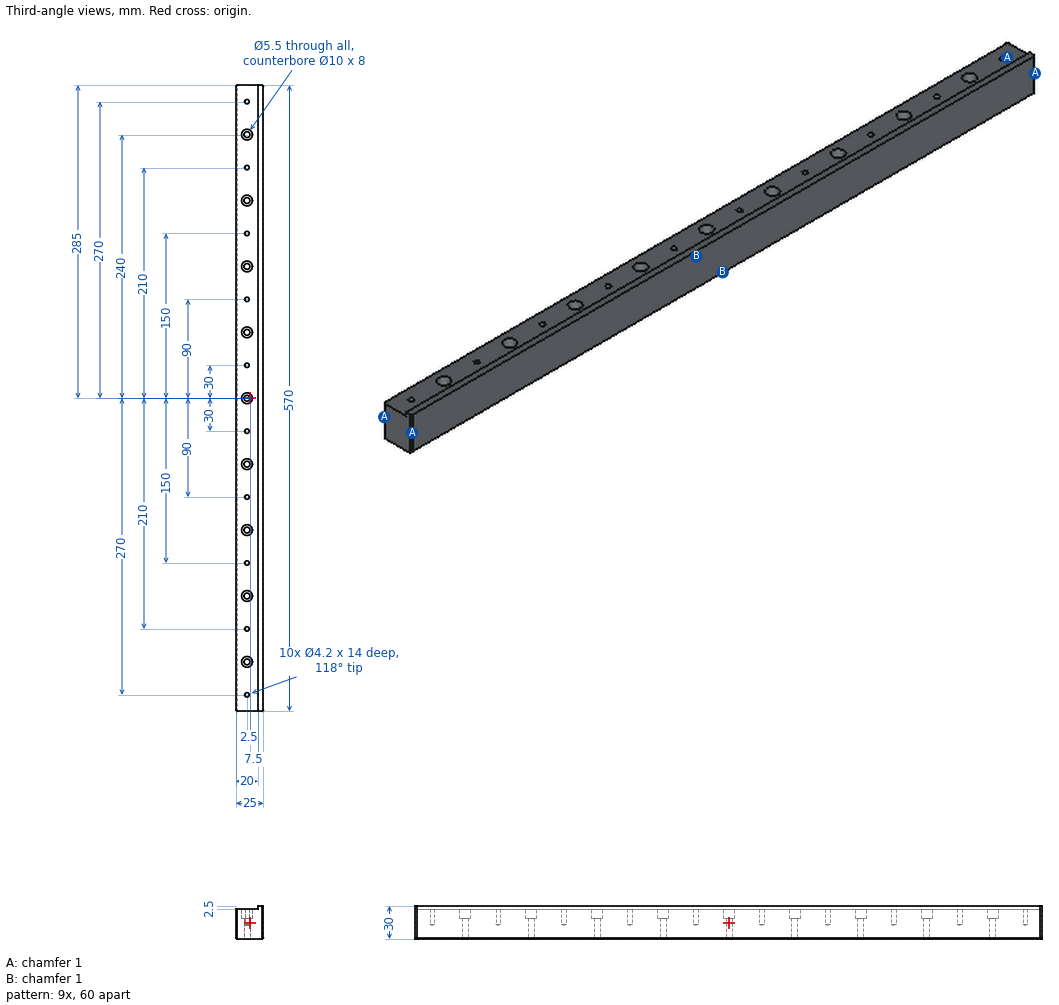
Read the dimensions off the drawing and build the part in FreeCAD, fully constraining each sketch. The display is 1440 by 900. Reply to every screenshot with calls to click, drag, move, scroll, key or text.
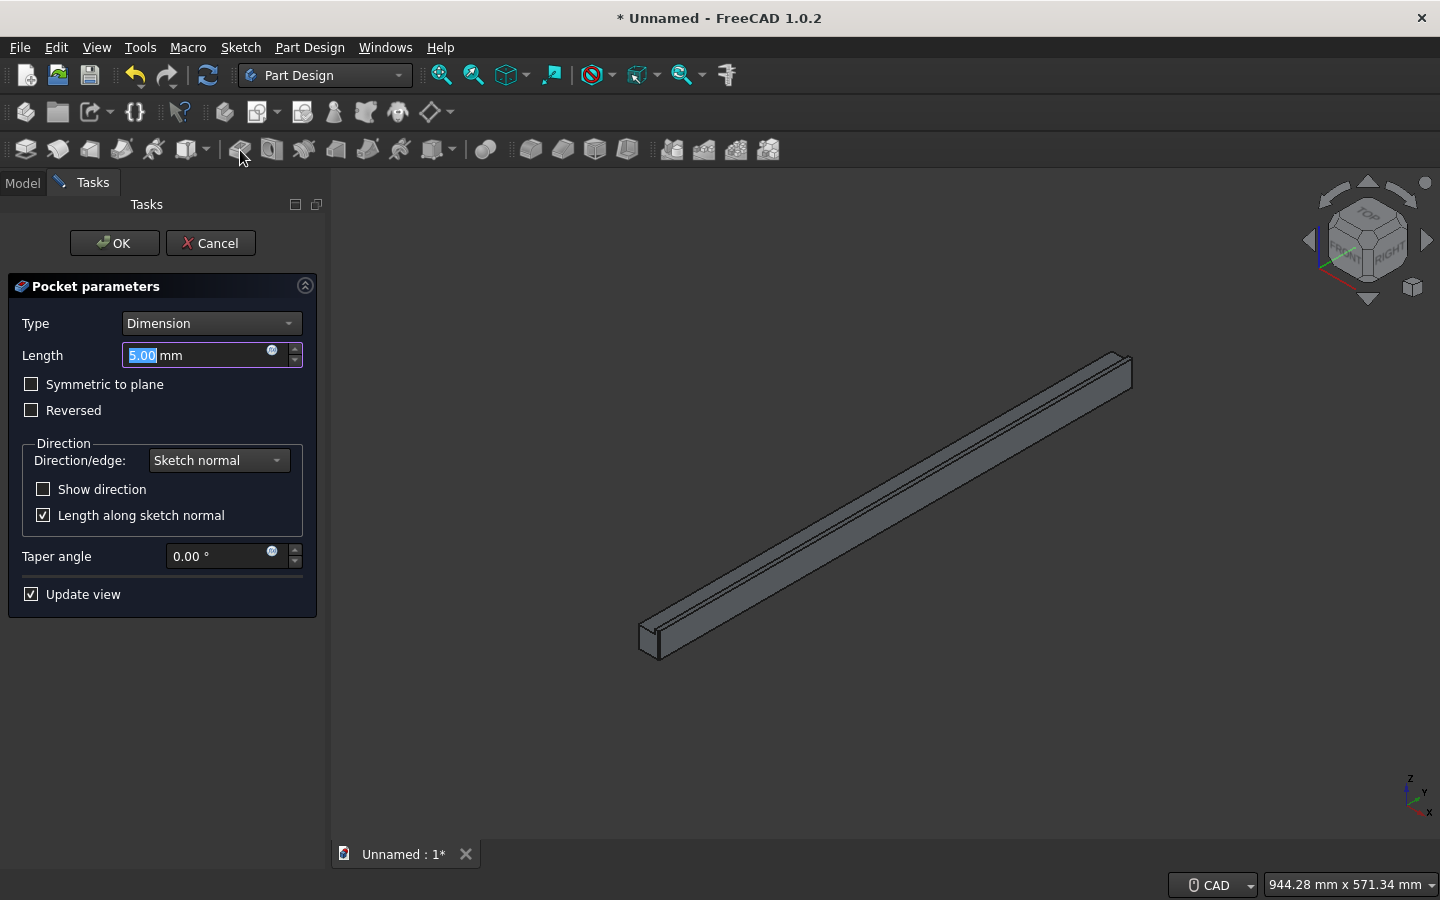
text(2.5)
key(Tab)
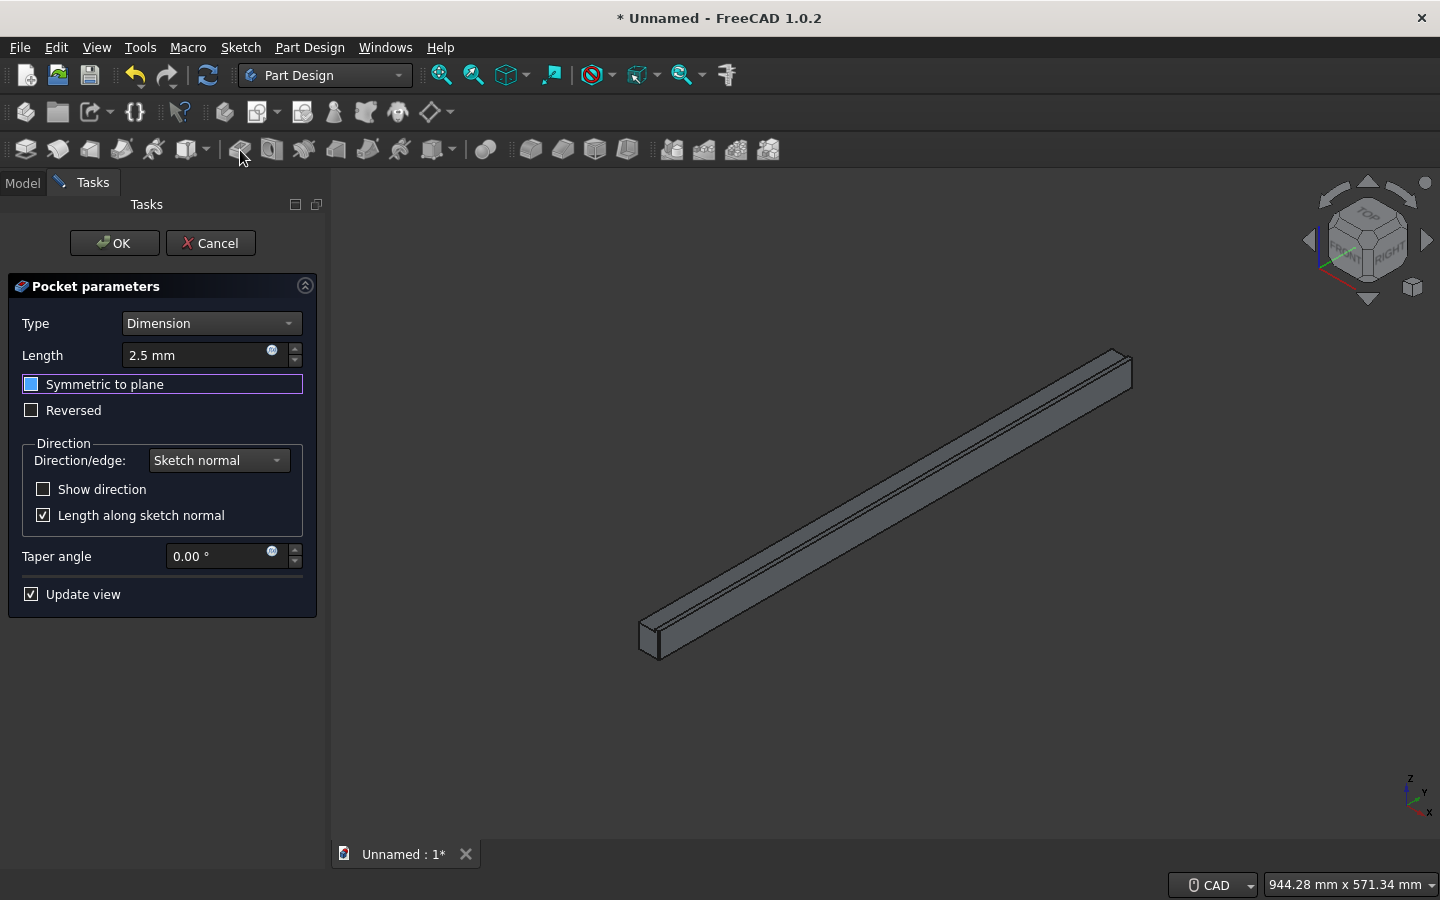
click(115, 243)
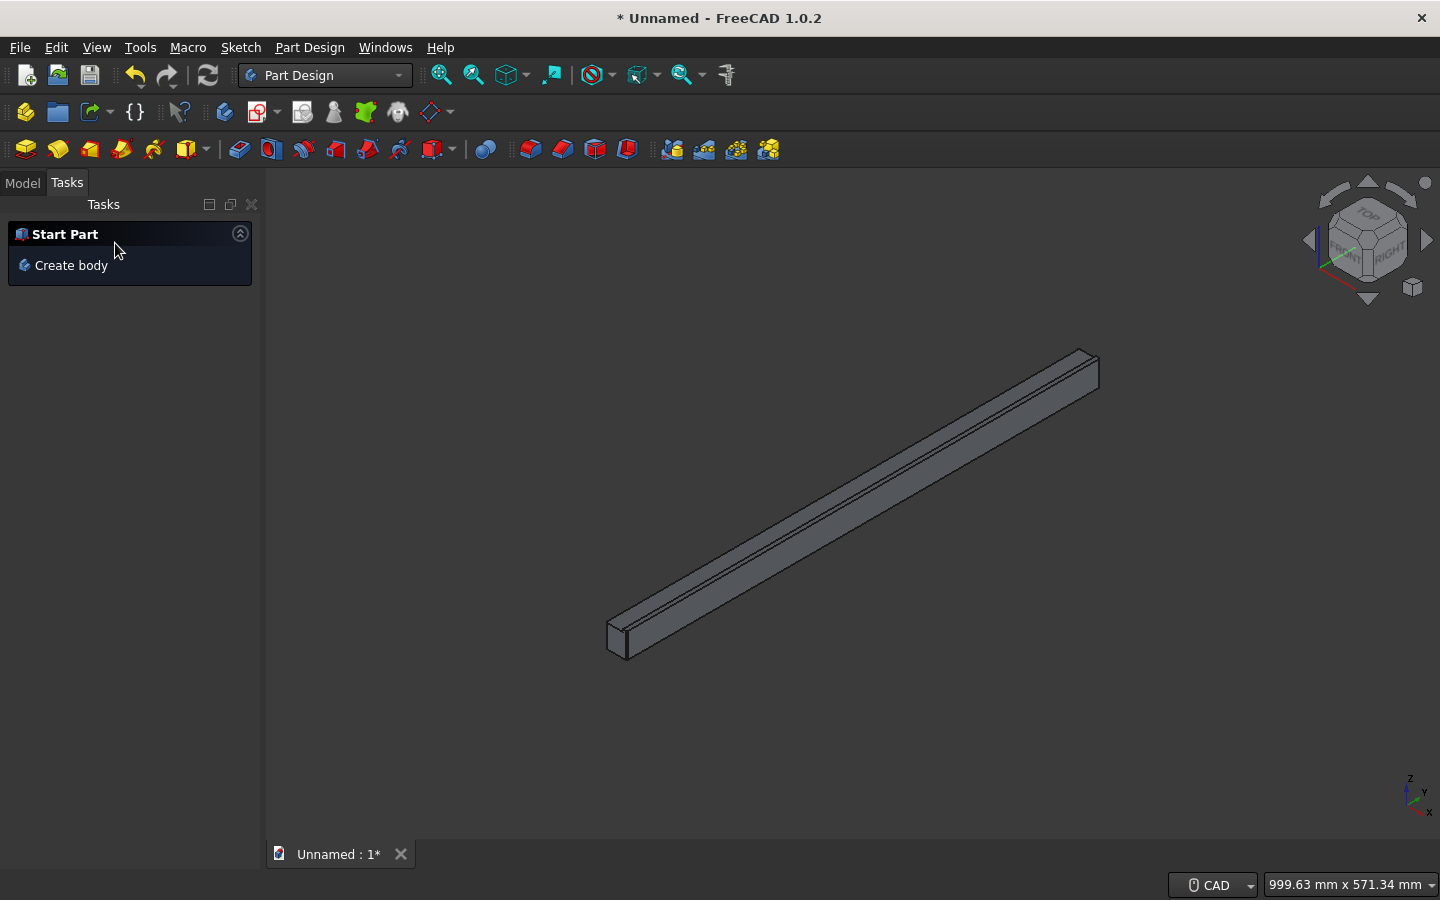
key(2)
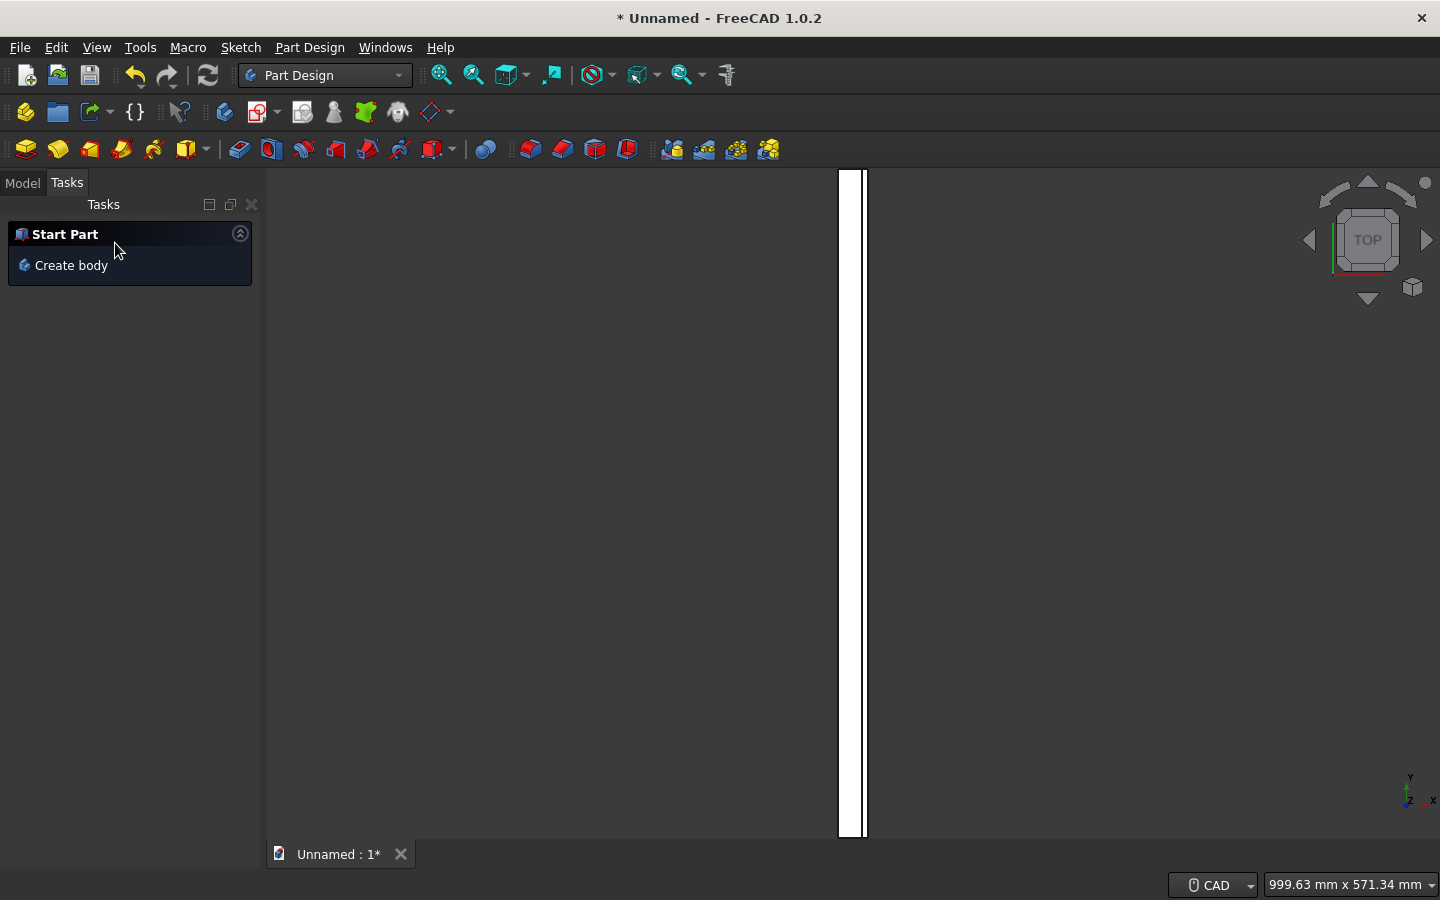
key(0)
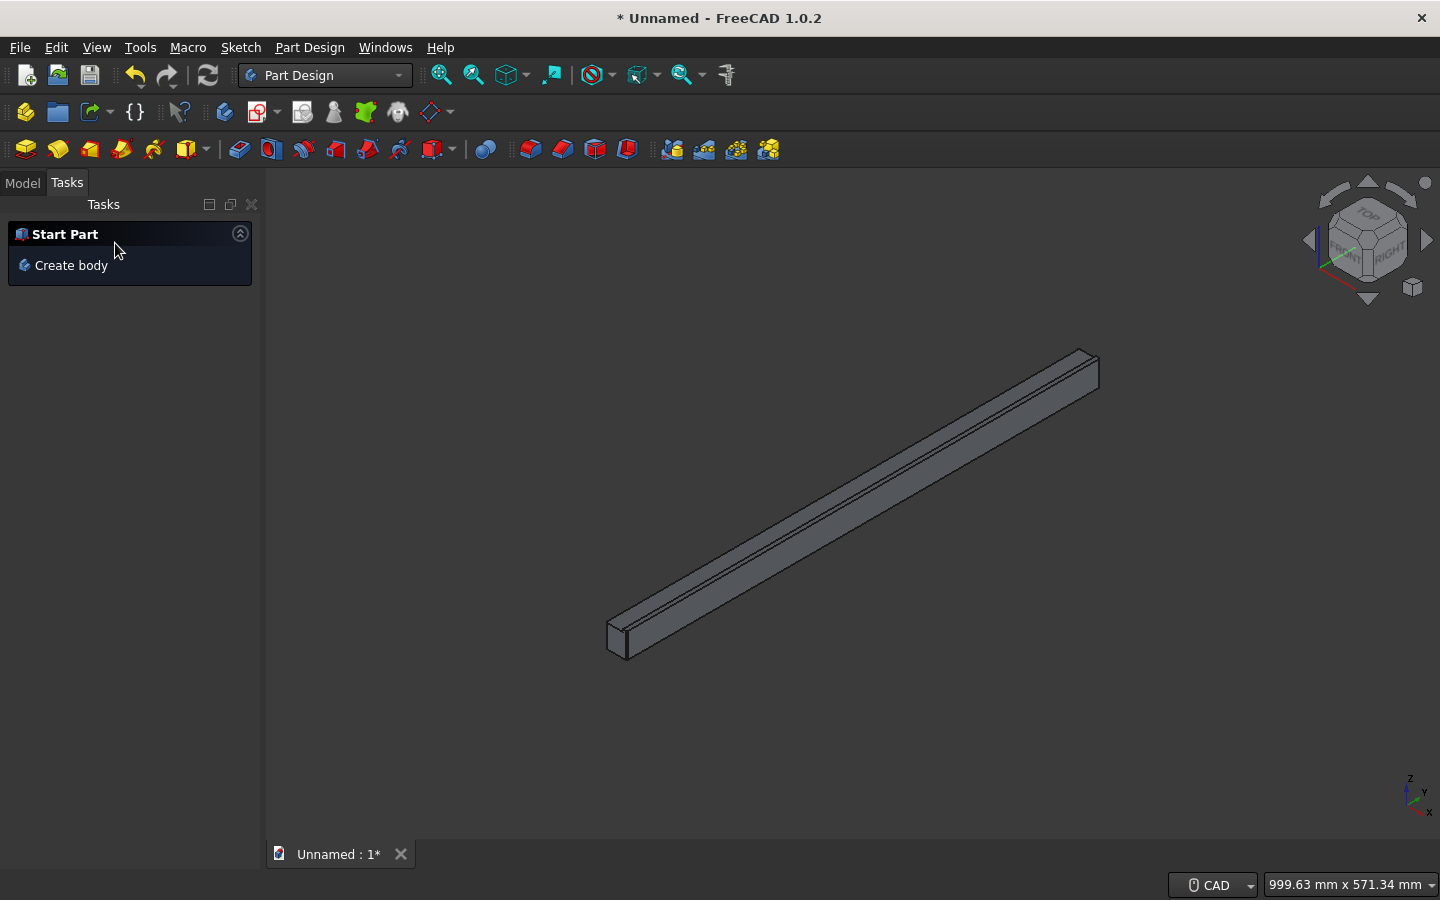
key(1)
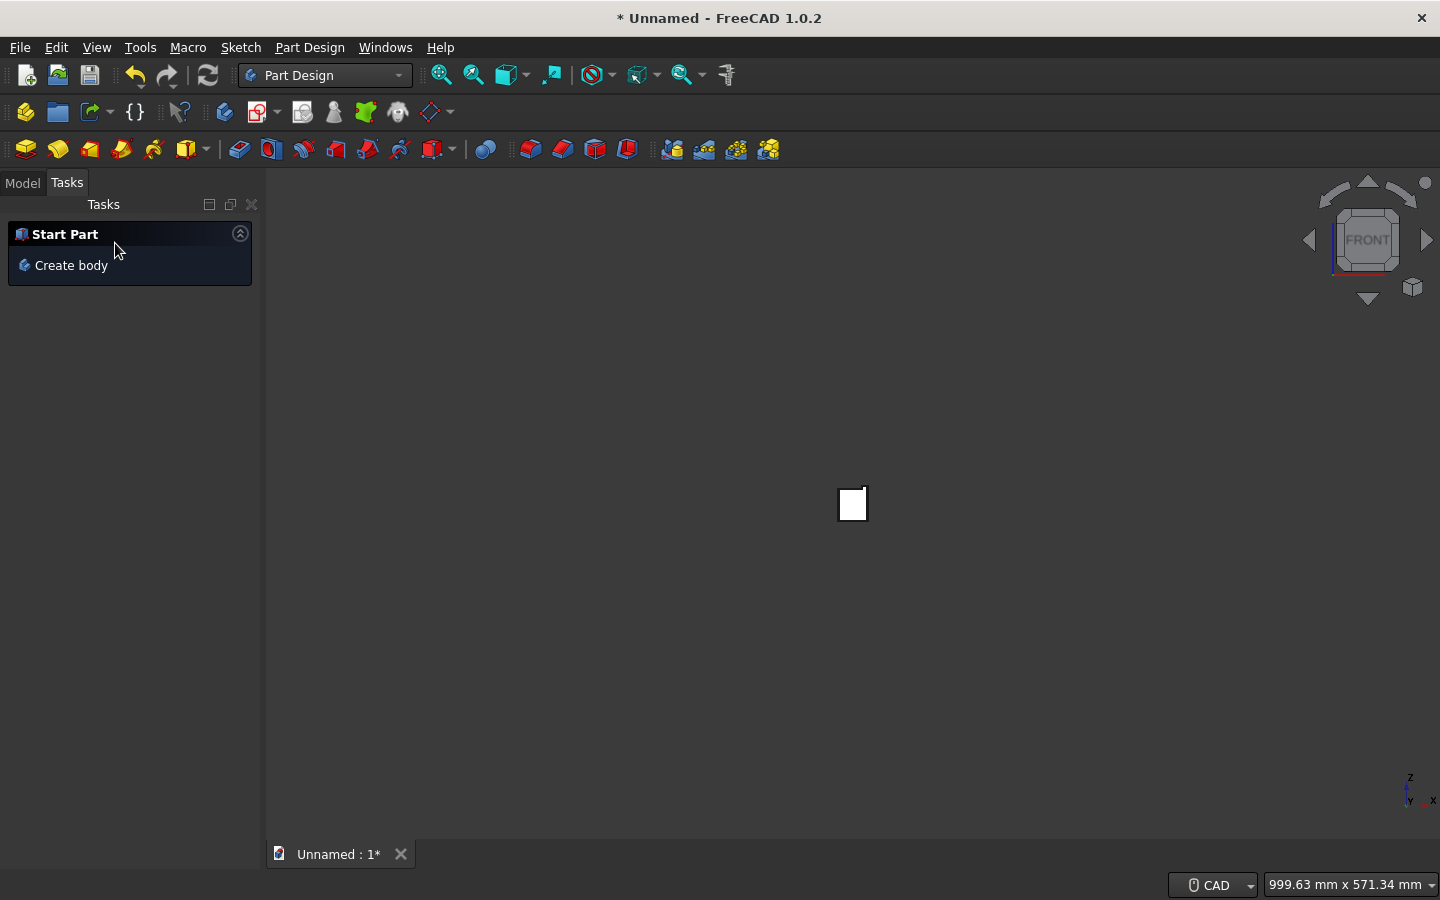
click(442, 76)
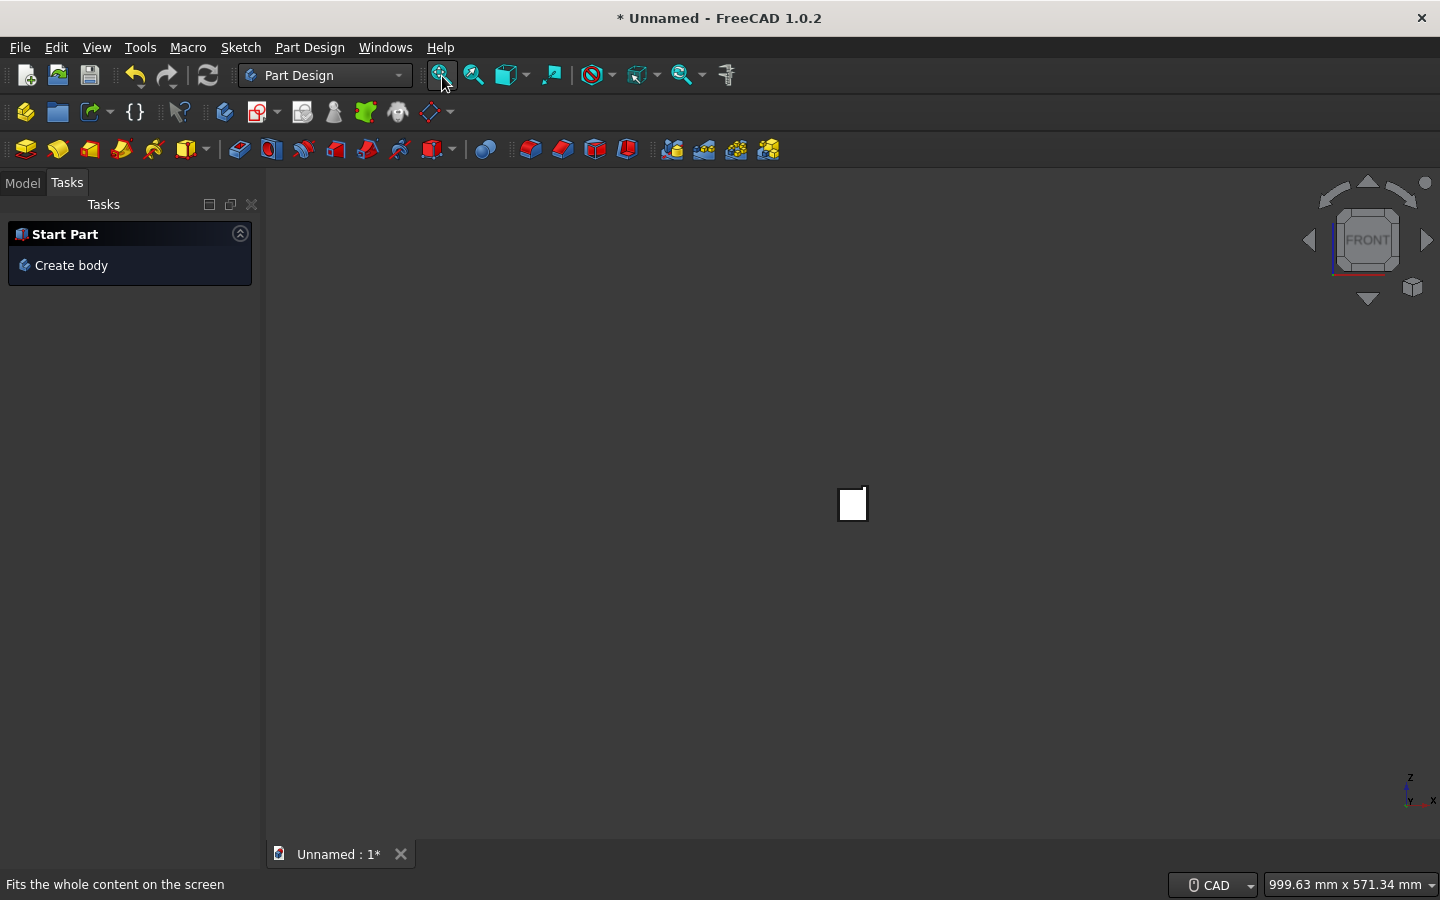
key(3)